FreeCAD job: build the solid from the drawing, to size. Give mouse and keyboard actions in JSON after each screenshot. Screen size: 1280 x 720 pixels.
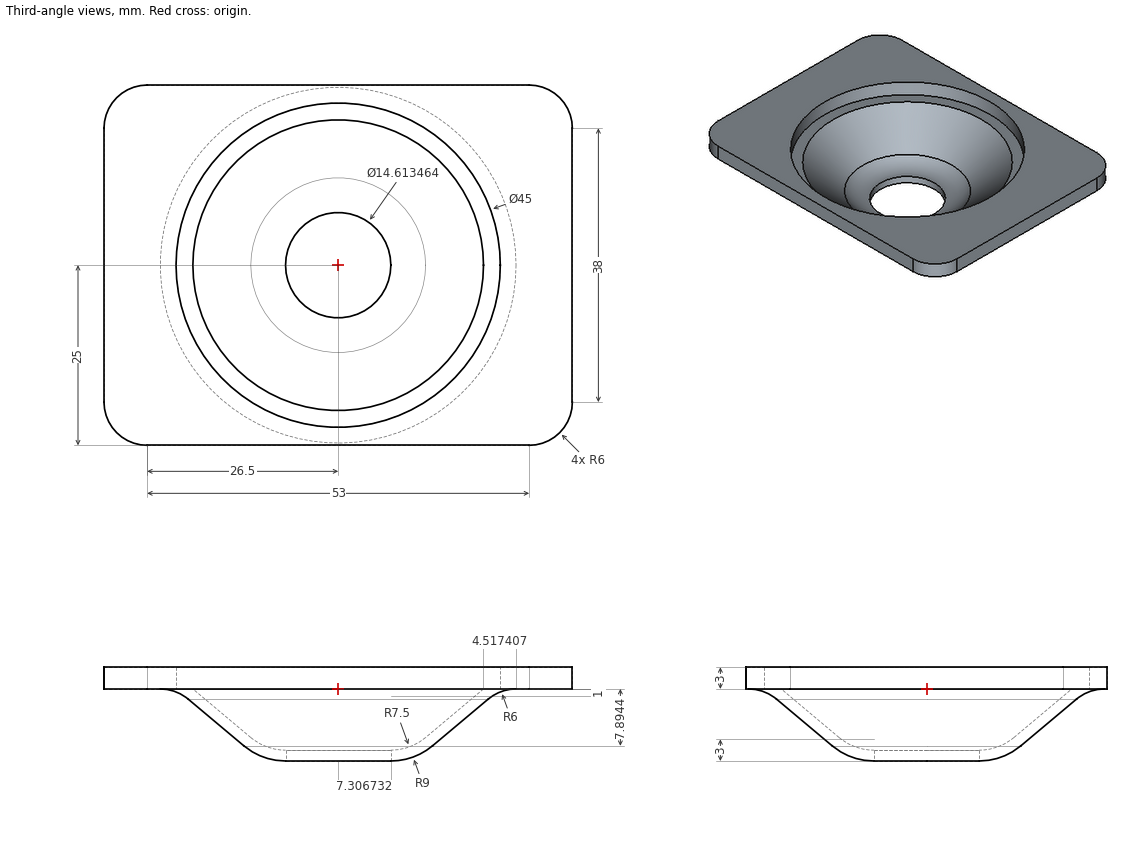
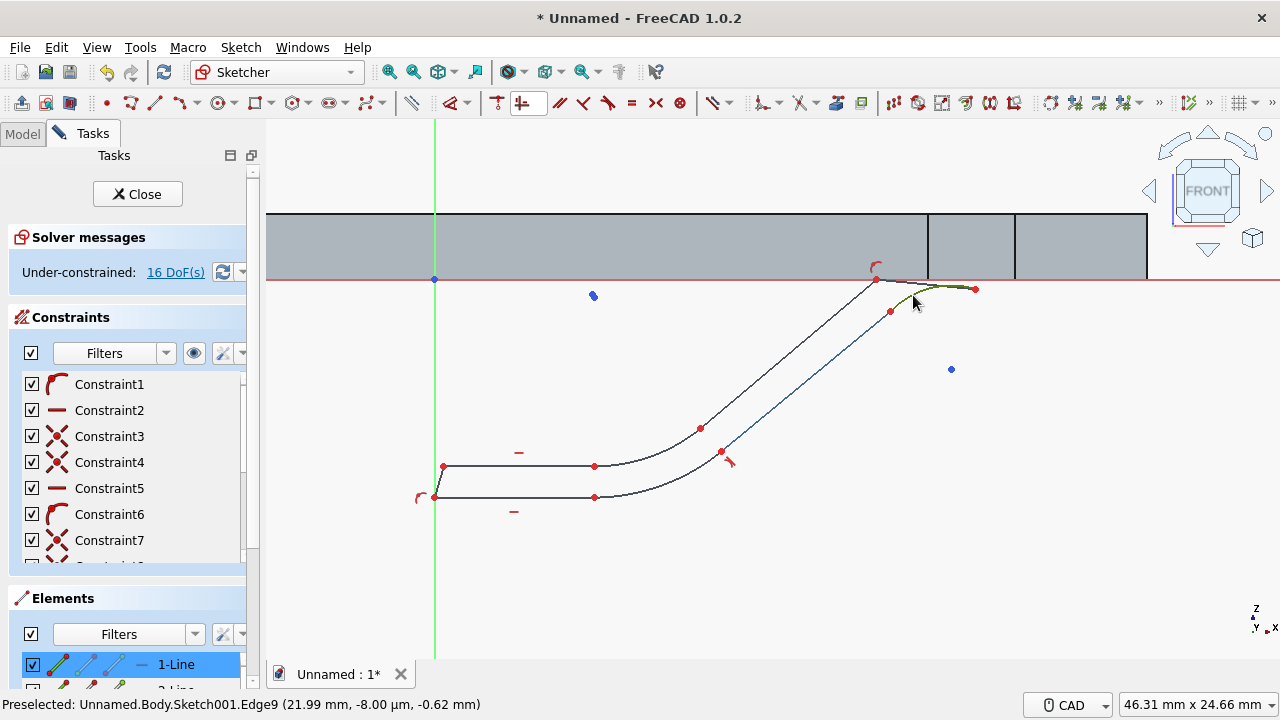
{"action": "left_click", "coordinate": [608, 104]}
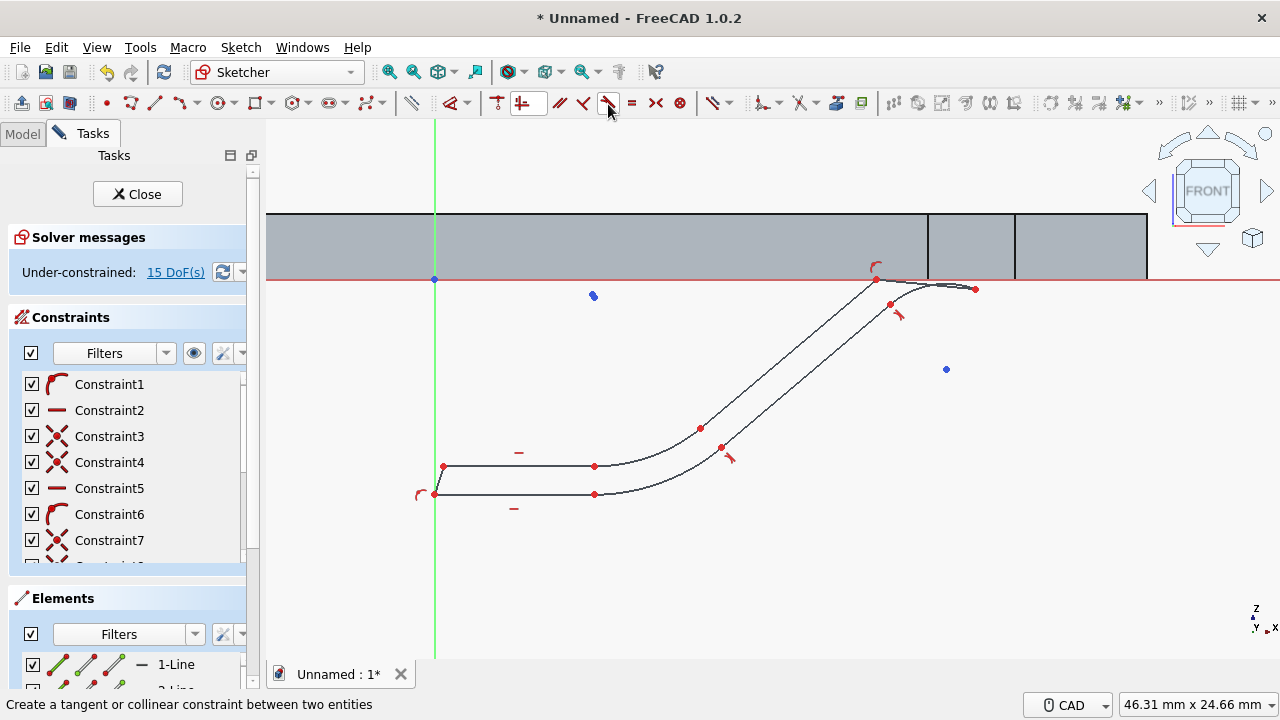
{"action": "left_click", "coordinate": [547, 495]}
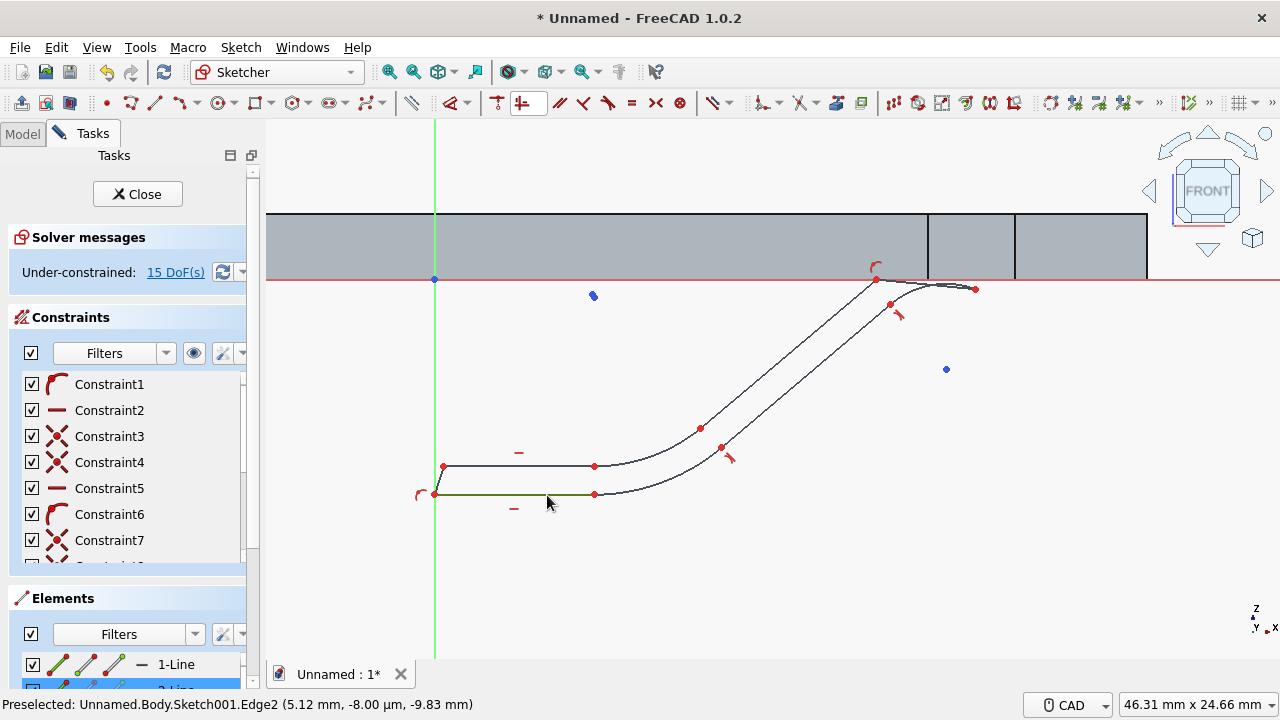
{"action": "left_click", "coordinate": [636, 490]}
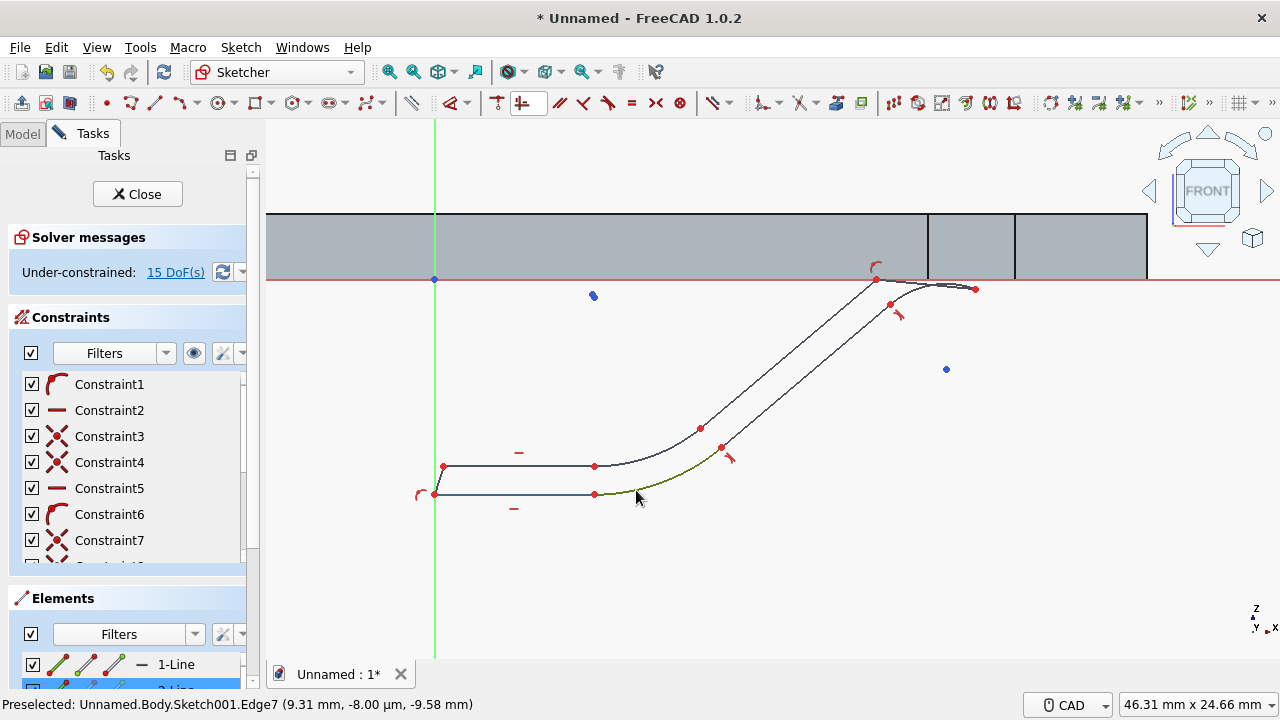
{"action": "left_click", "coordinate": [608, 104]}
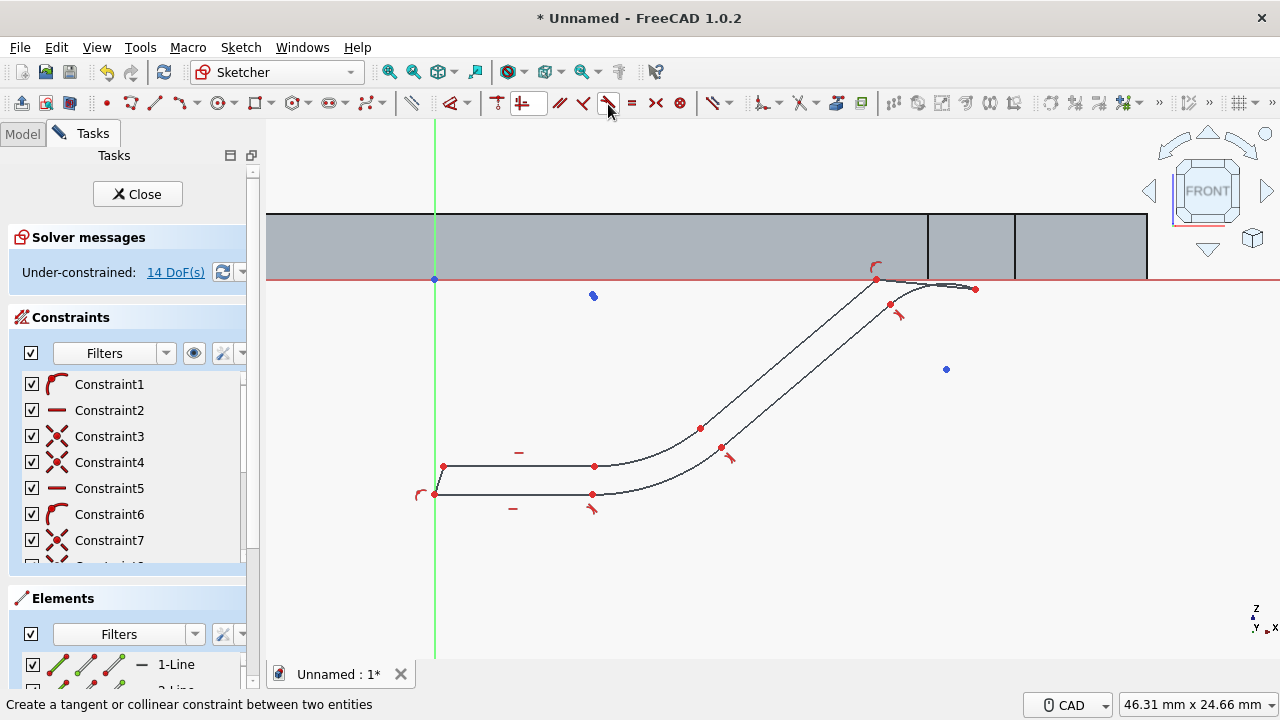
{"action": "left_click", "coordinate": [489, 466]}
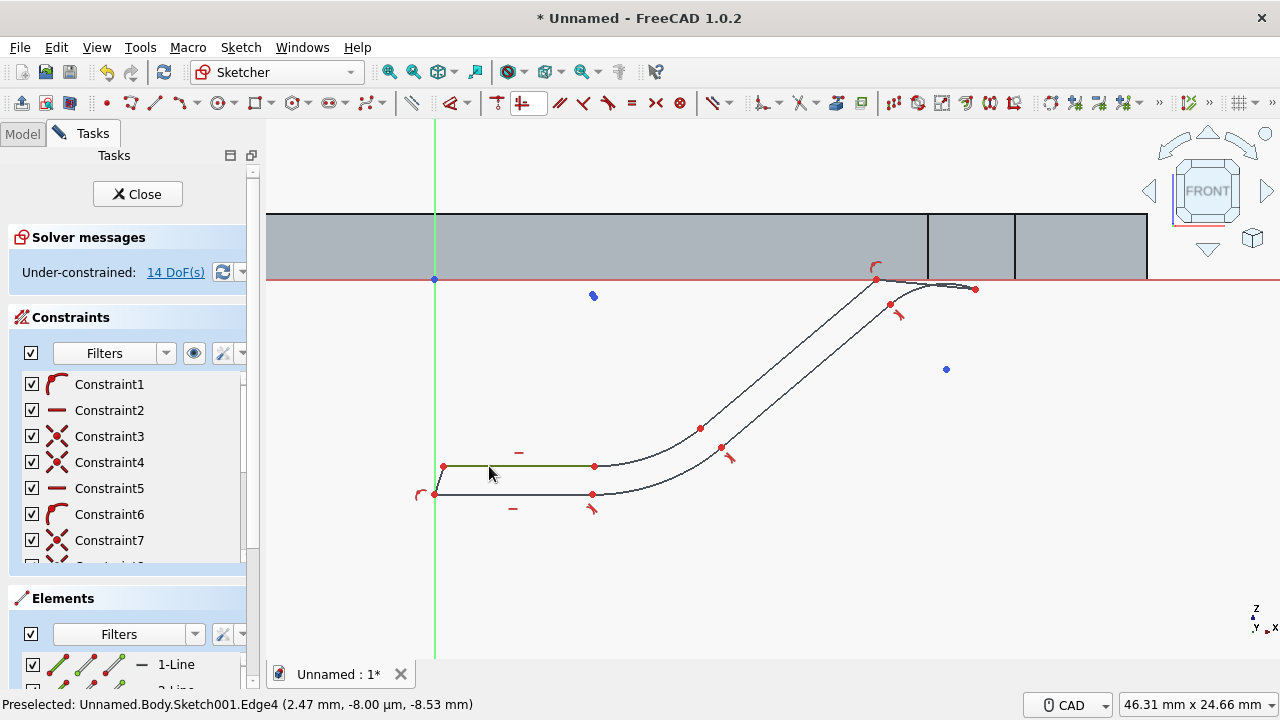
{"action": "left_click", "coordinate": [629, 463]}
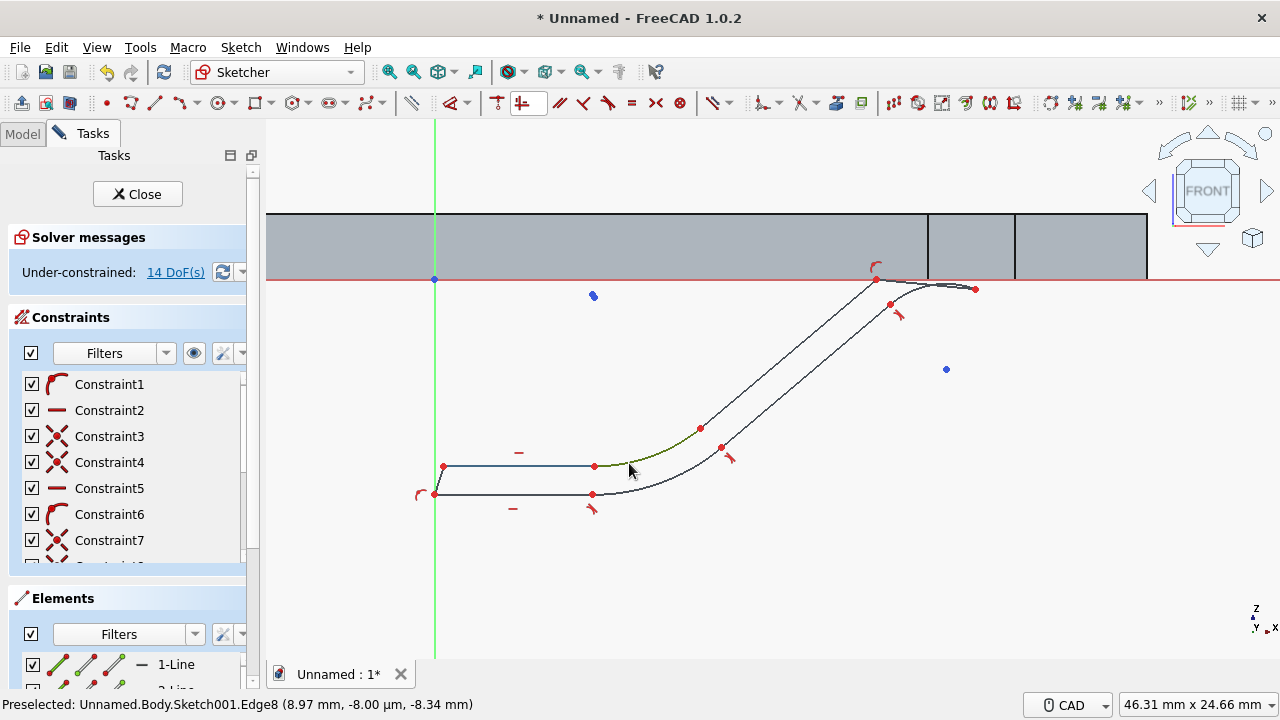
{"action": "key", "text": "t"}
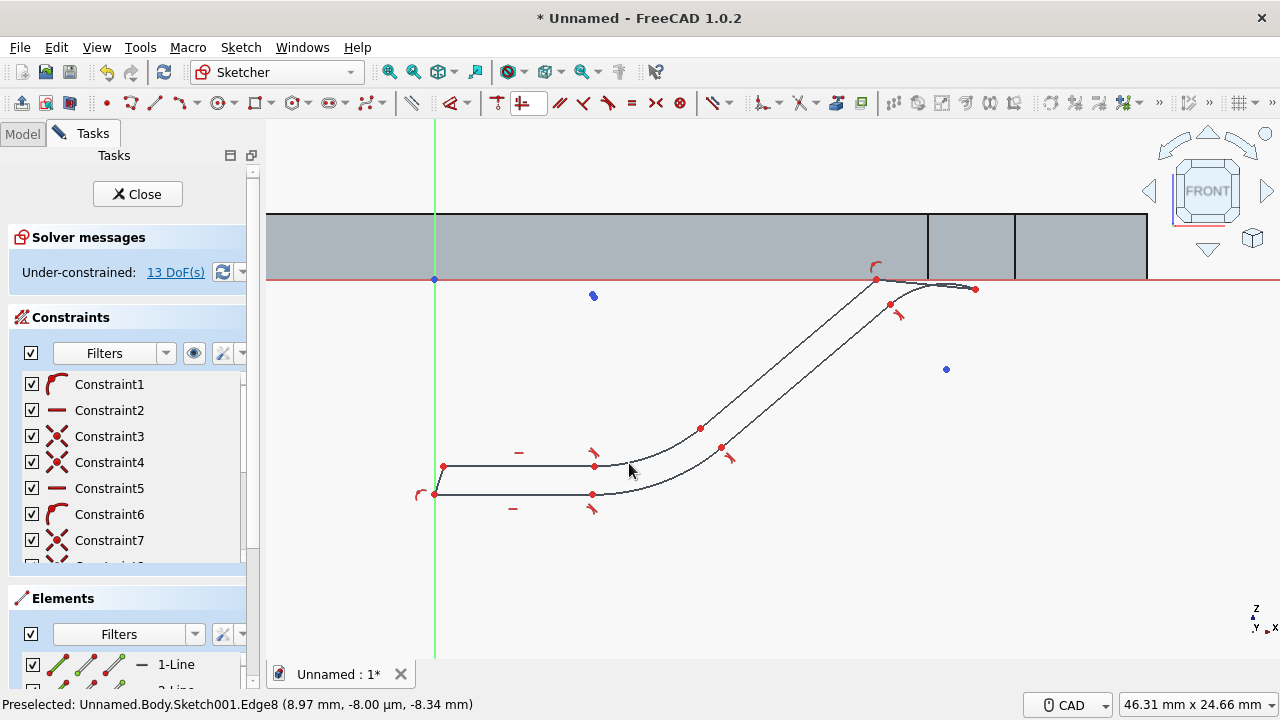
{"action": "left_click", "coordinate": [754, 384]}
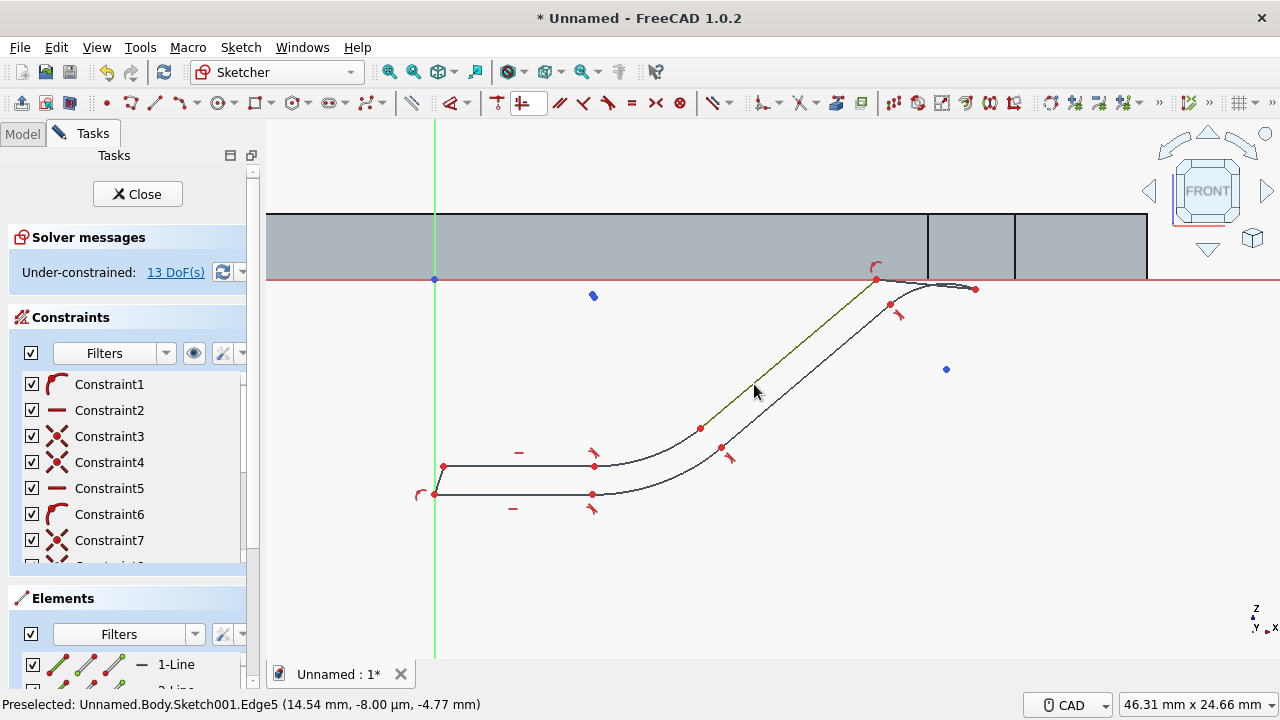
{"action": "left_click", "coordinate": [629, 463]}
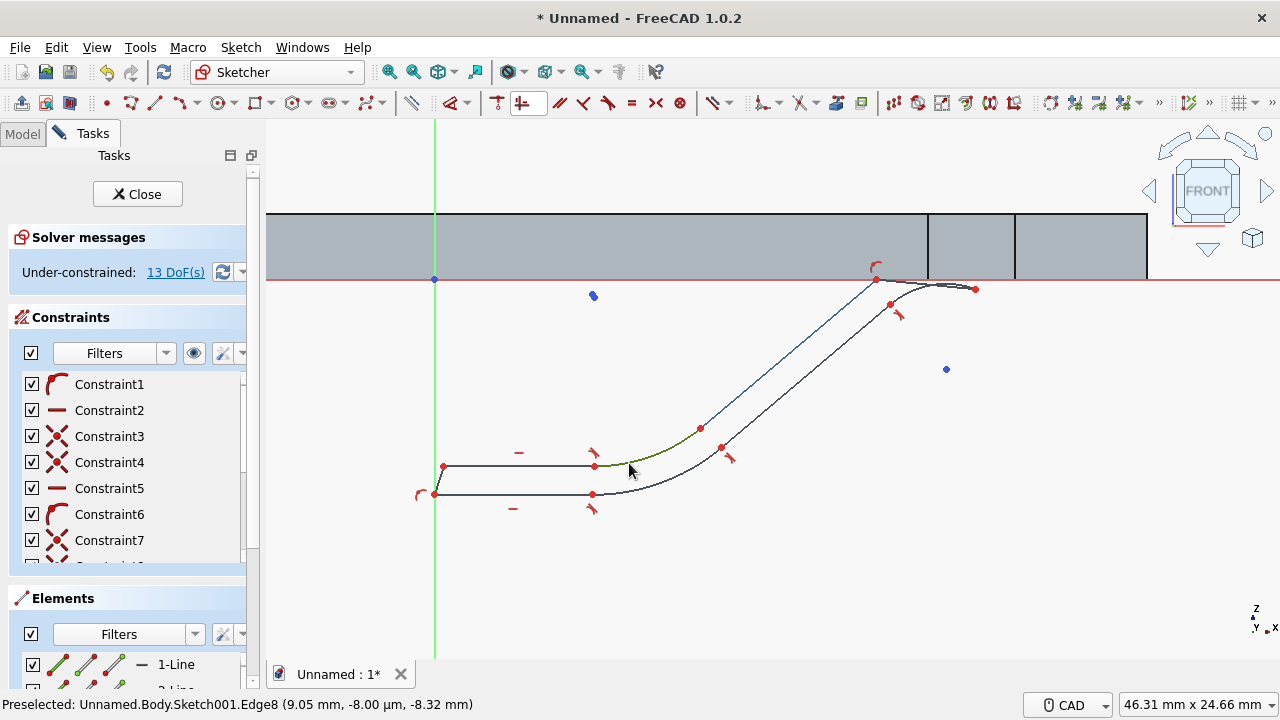
{"action": "key", "text": "t"}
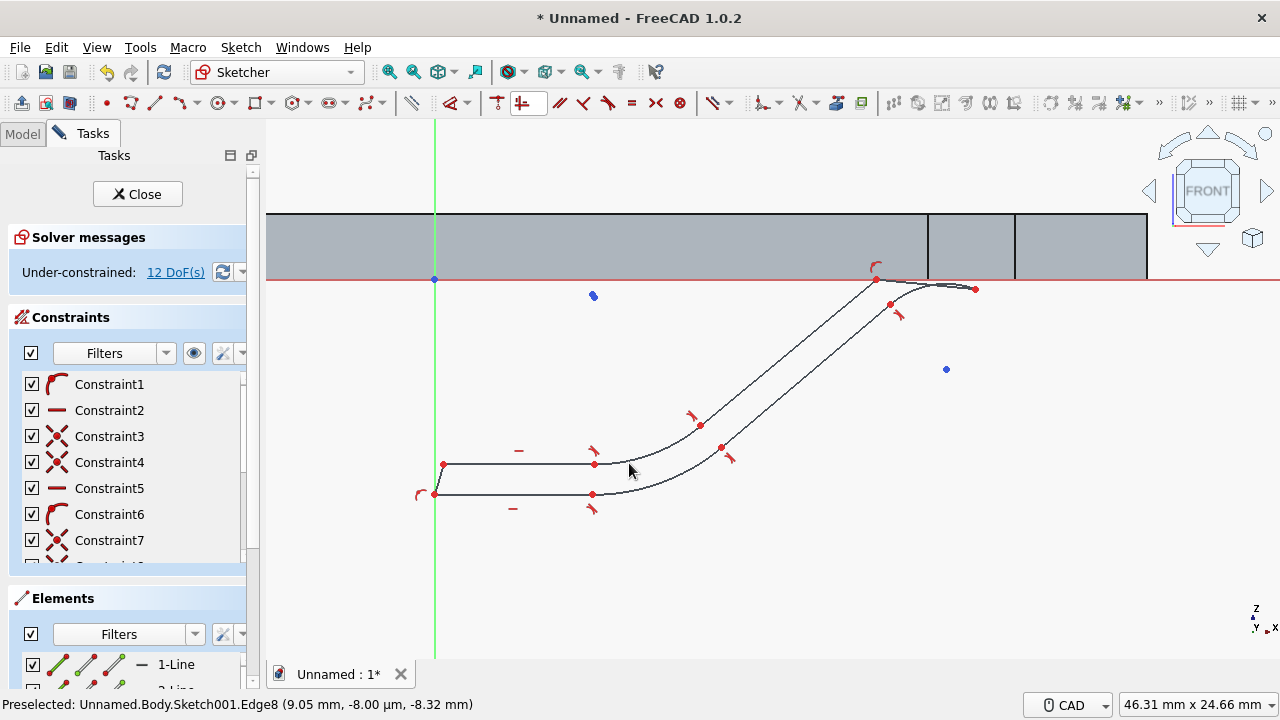
{"action": "scroll", "coordinate": [907, 283], "scroll_direction": "up", "scroll_amount": 2}